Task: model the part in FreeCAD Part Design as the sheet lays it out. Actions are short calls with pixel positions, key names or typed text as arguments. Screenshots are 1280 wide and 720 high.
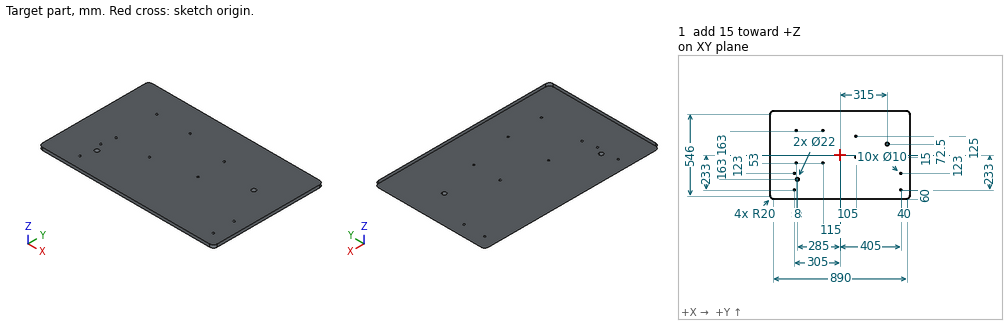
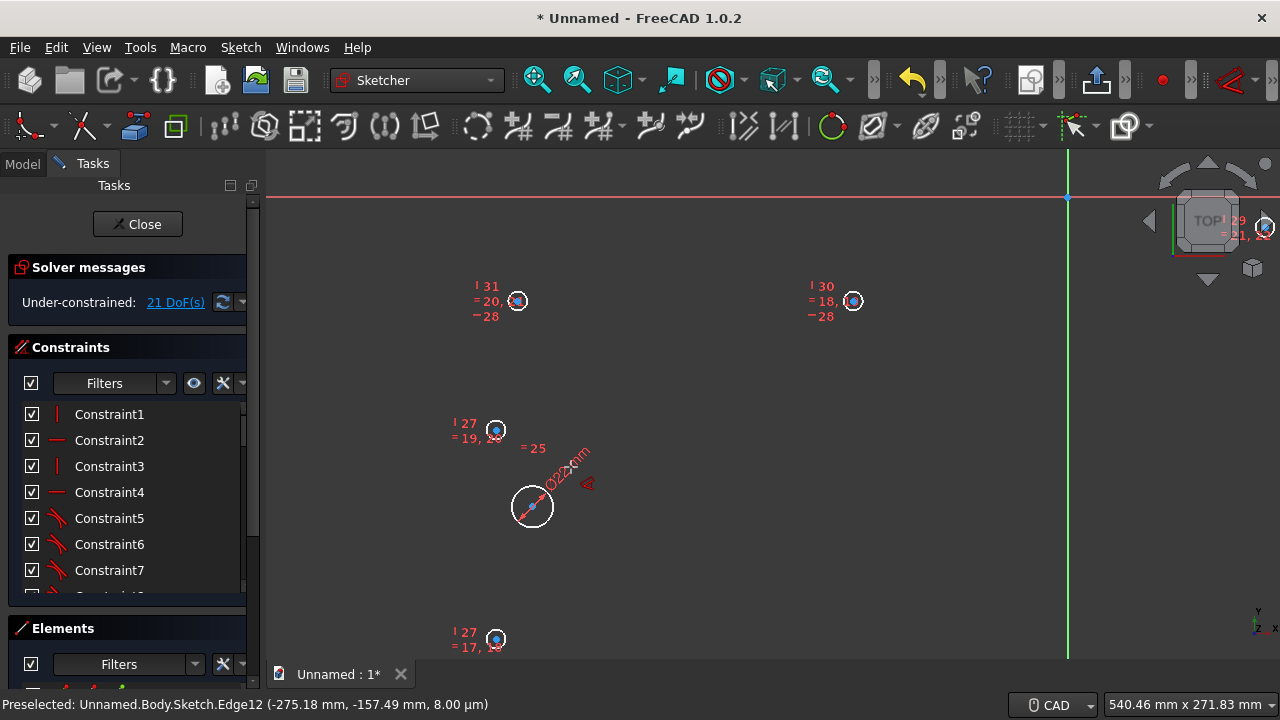
click(853, 301)
click(819, 249)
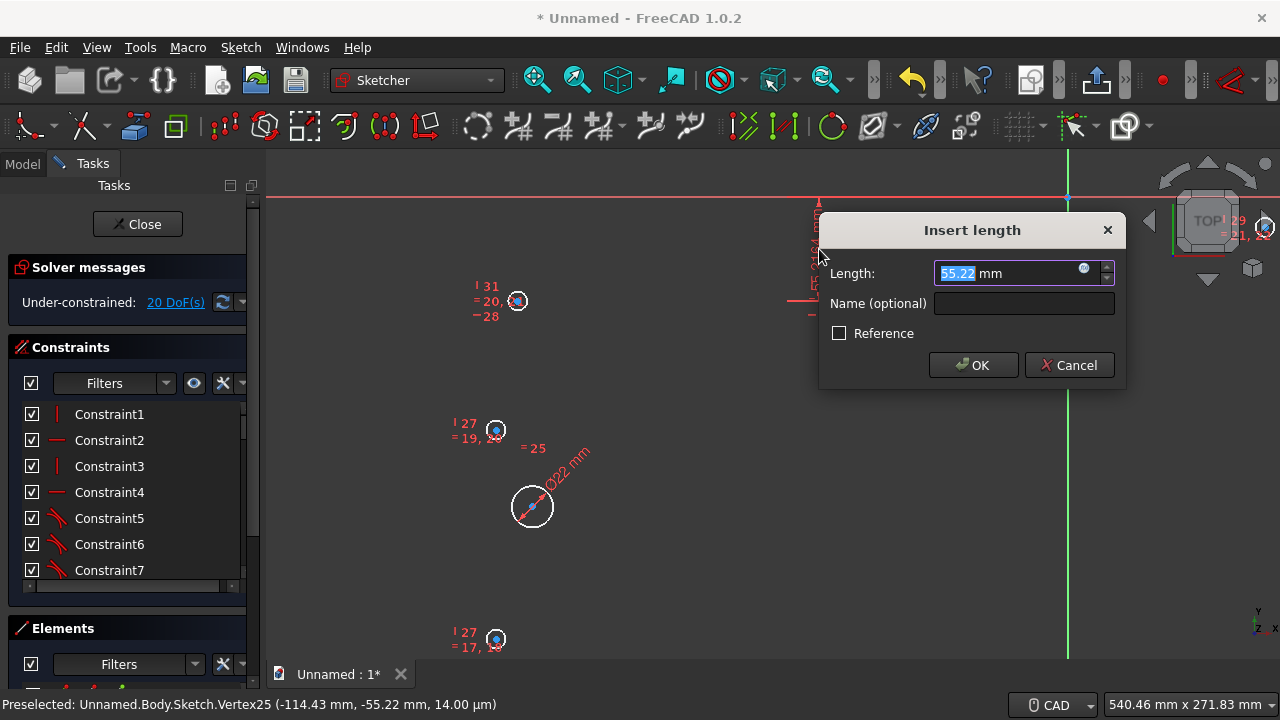
text(53)
key(Return)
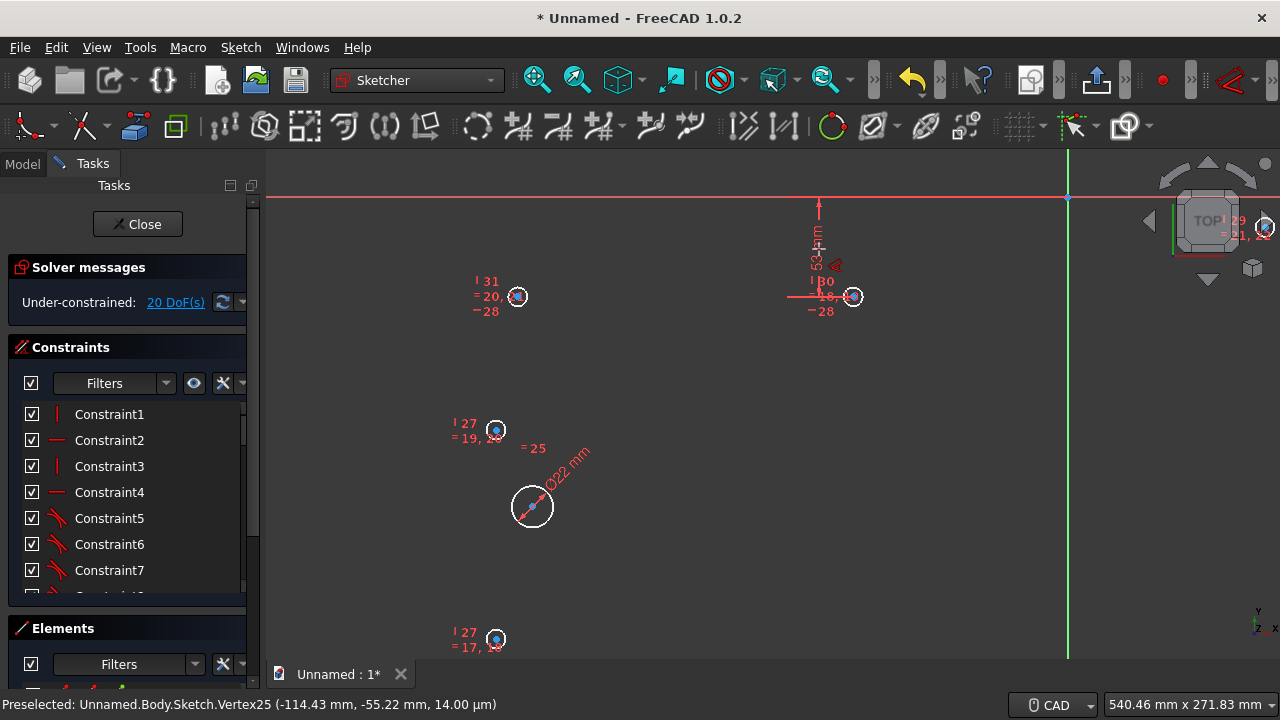
scroll(548, 493, down, 6)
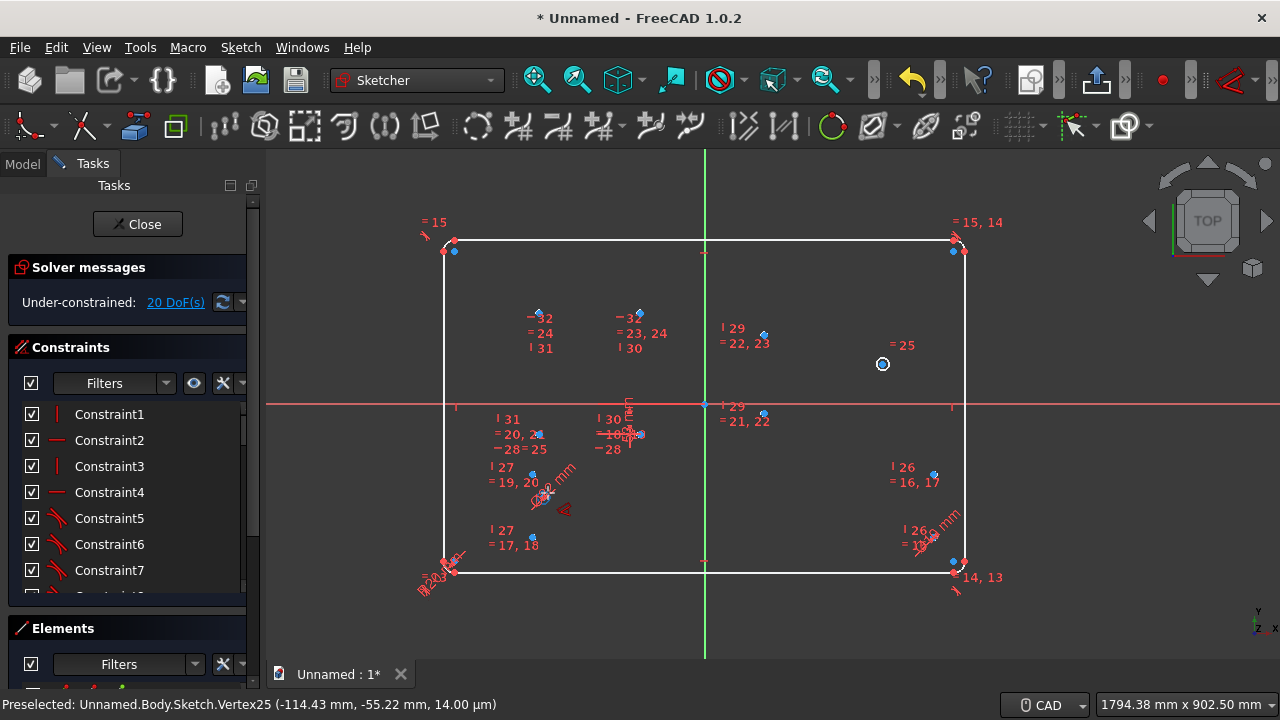
scroll(764, 413, up, 8)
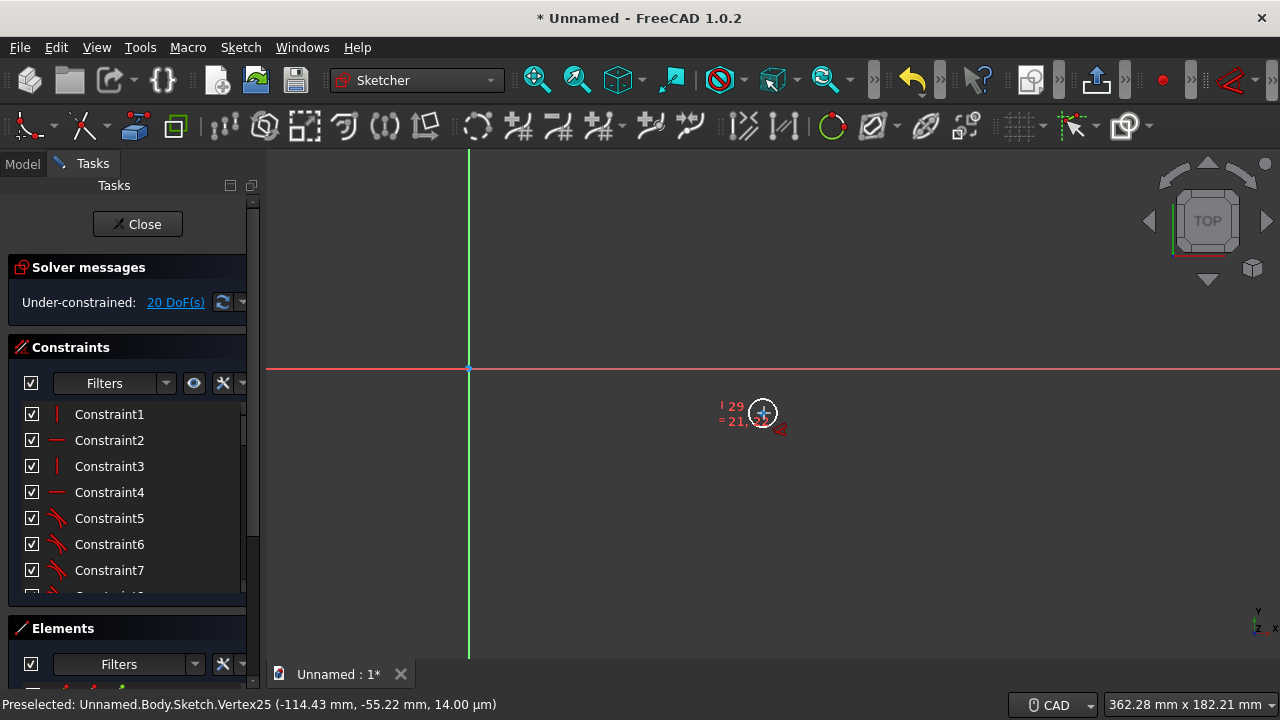
click(763, 413)
click(797, 391)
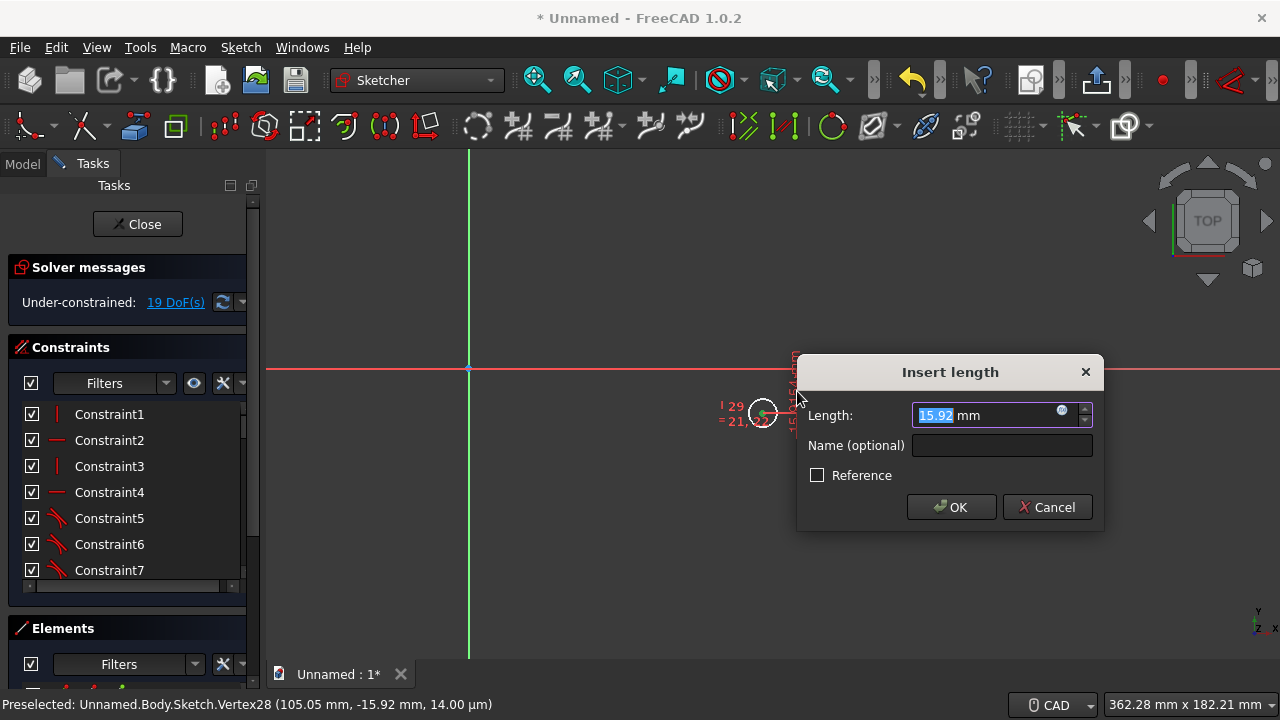
text(15)
key(Return)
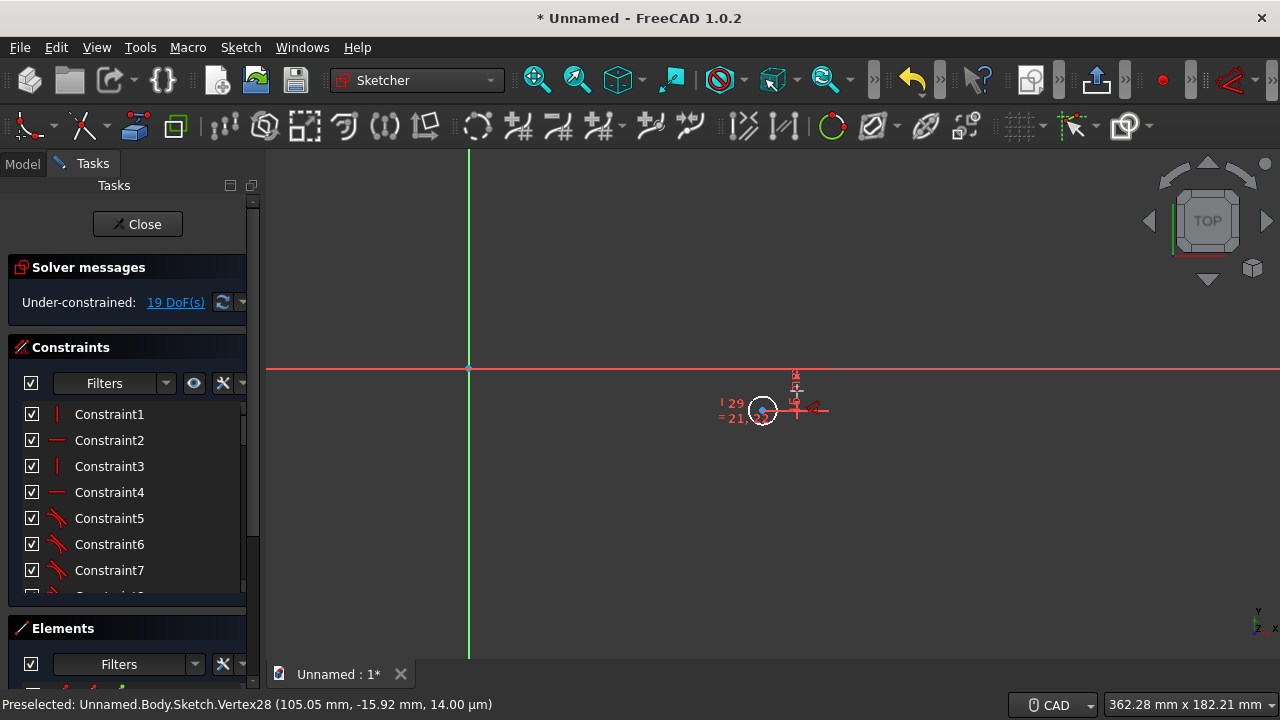
scroll(764, 413, down, 8)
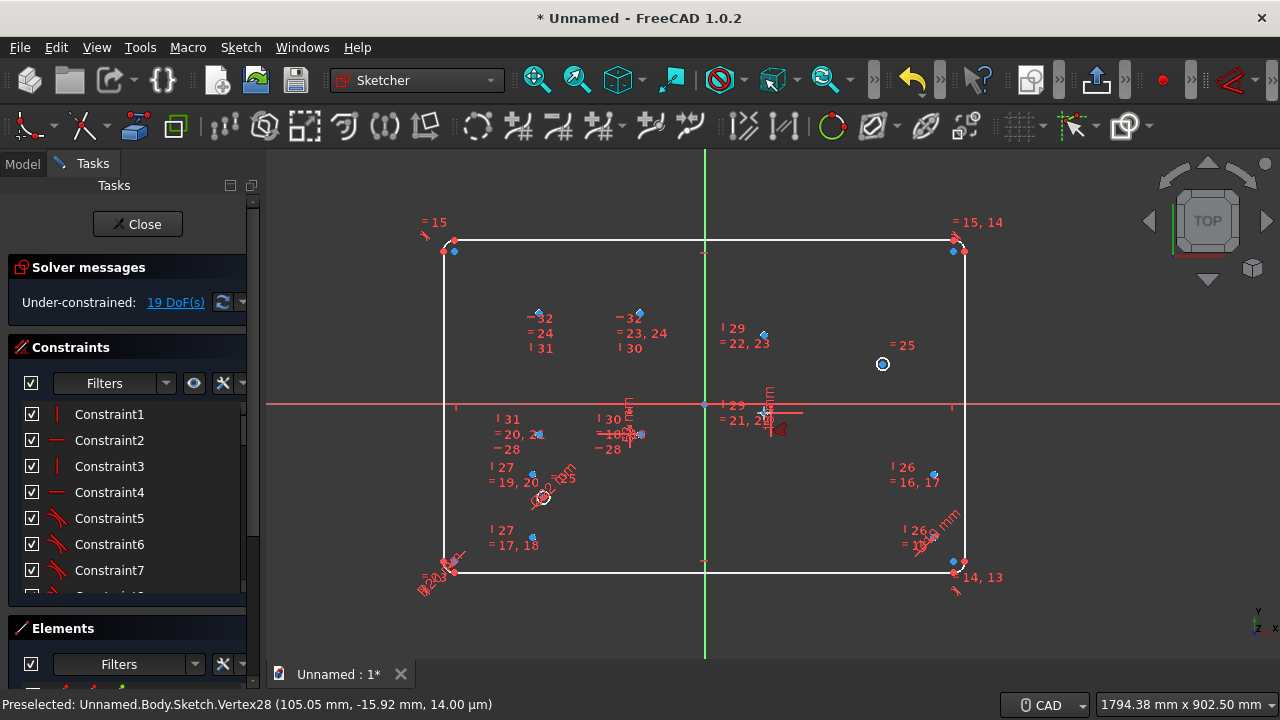
scroll(544, 498, up, 11)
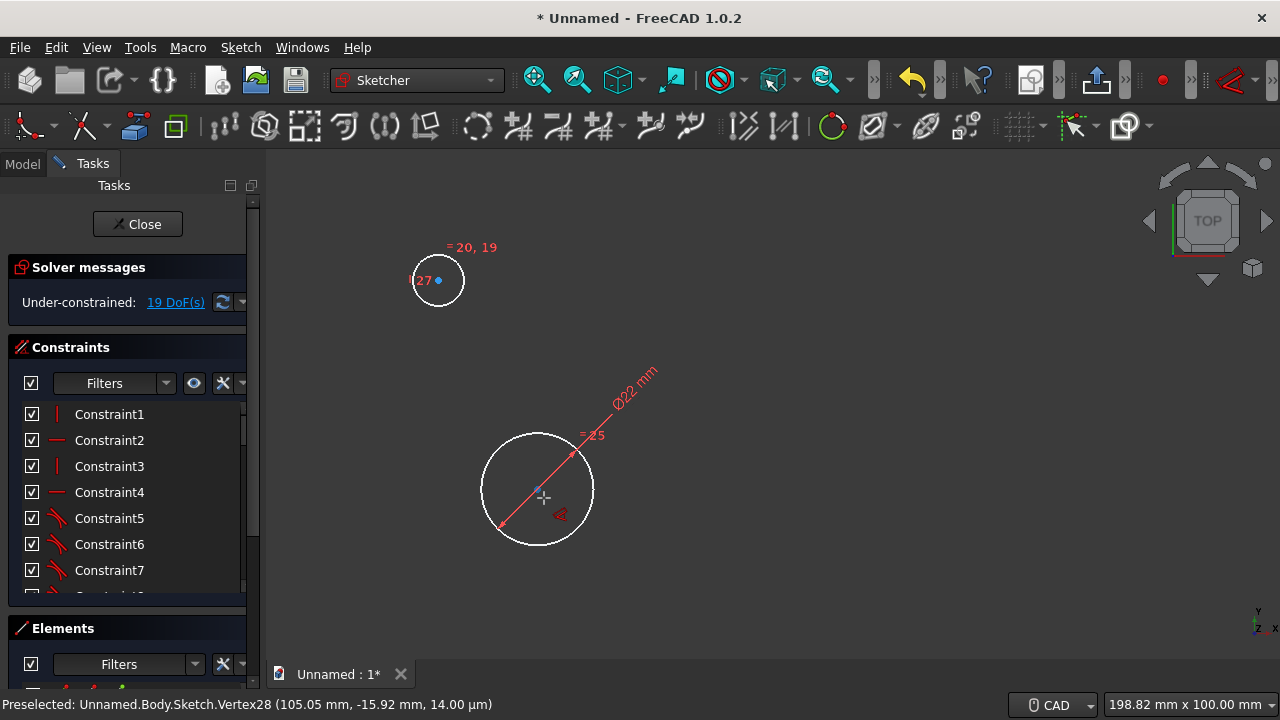
click(537, 489)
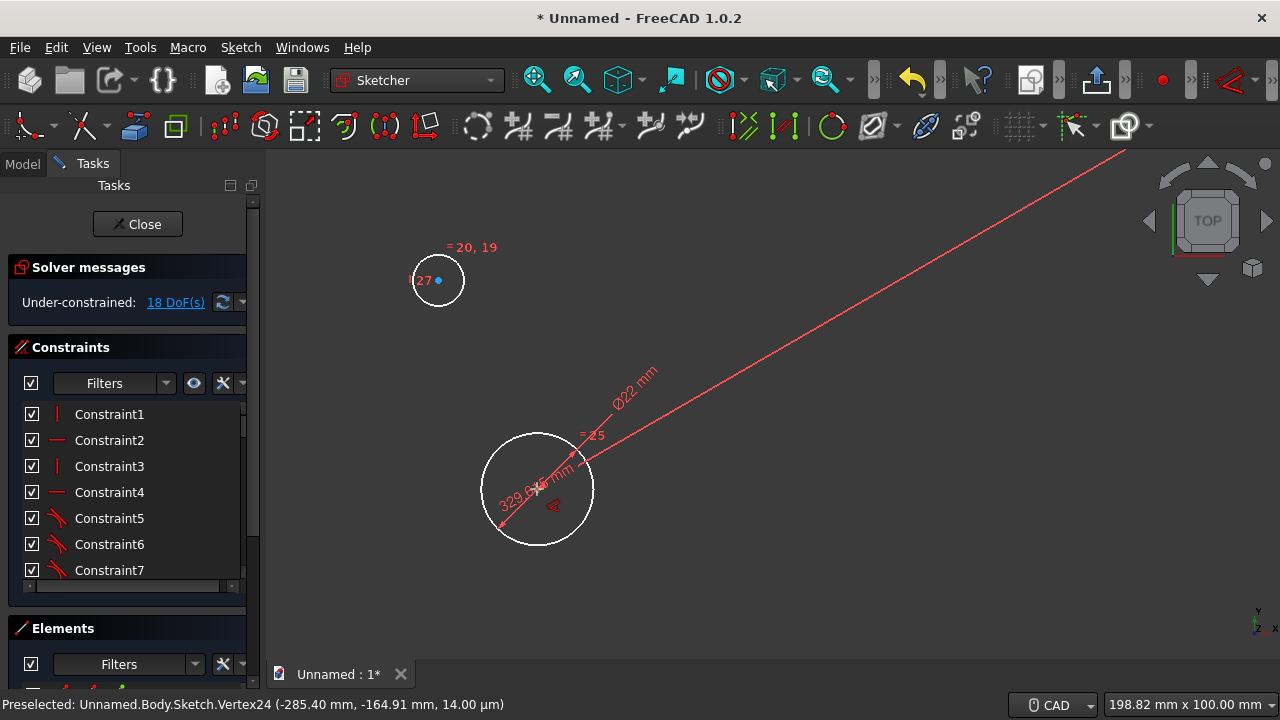
scroll(544, 498, down, 11)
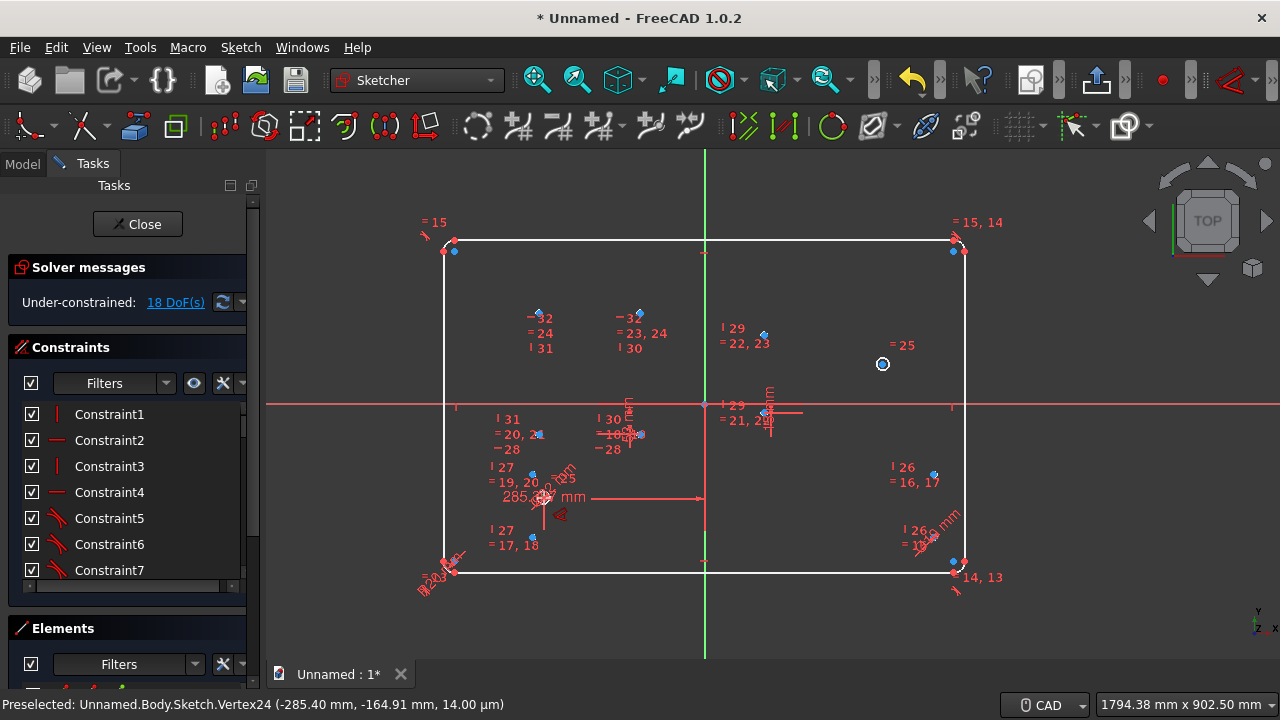
scroll(539, 434, up, 11)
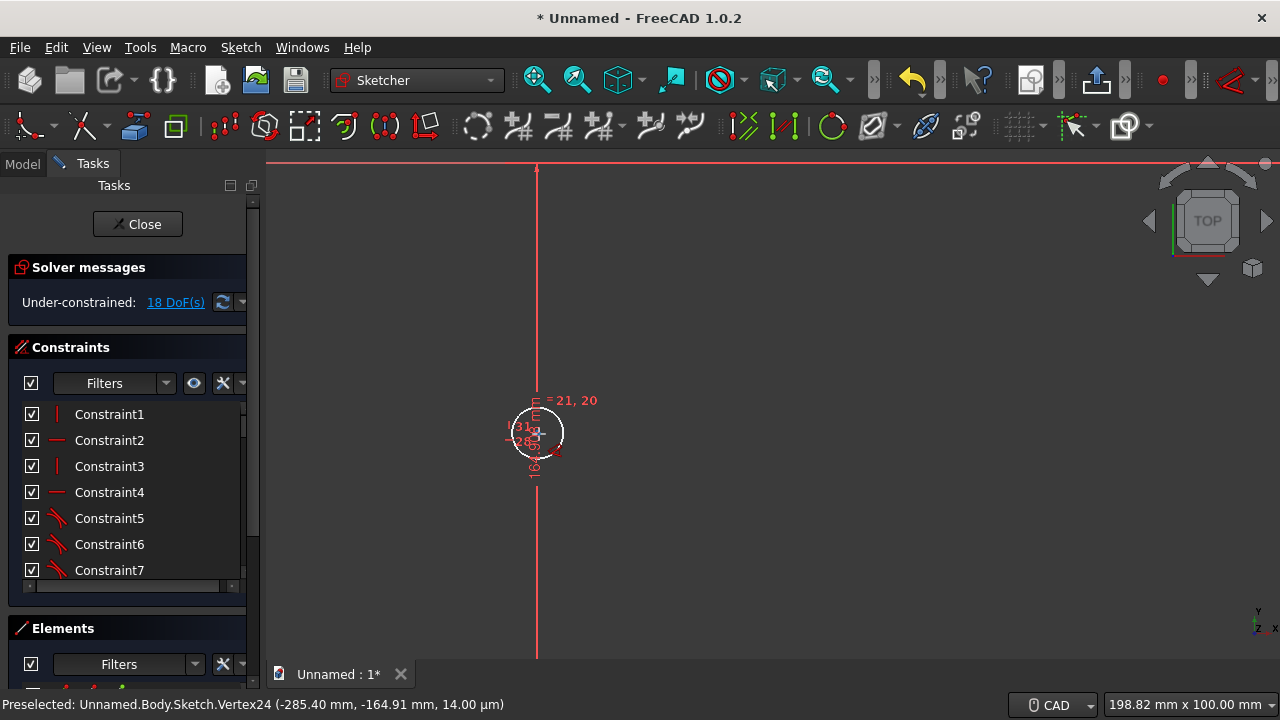
click(538, 433)
click(558, 399)